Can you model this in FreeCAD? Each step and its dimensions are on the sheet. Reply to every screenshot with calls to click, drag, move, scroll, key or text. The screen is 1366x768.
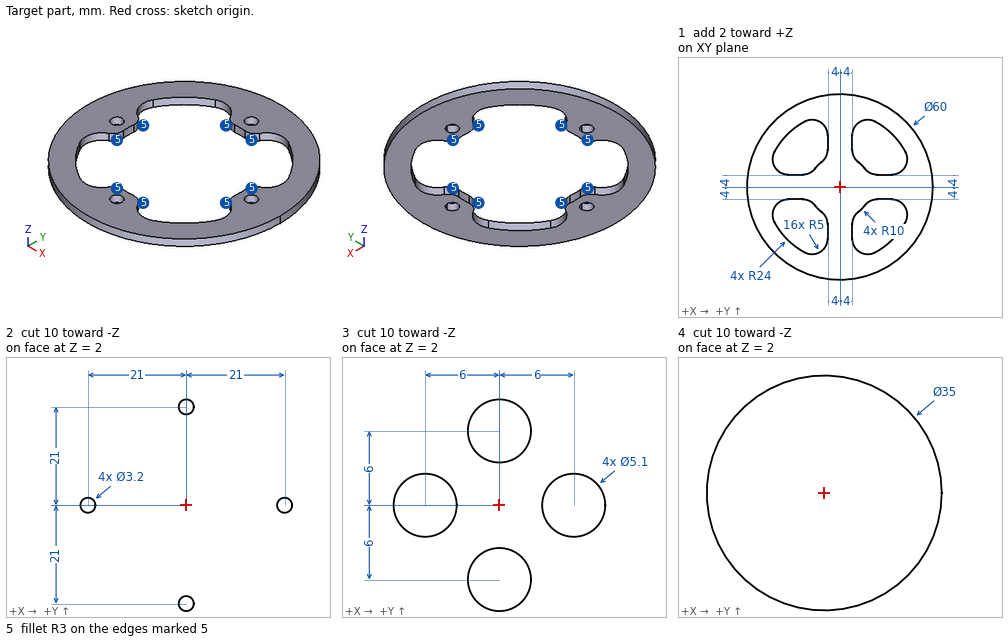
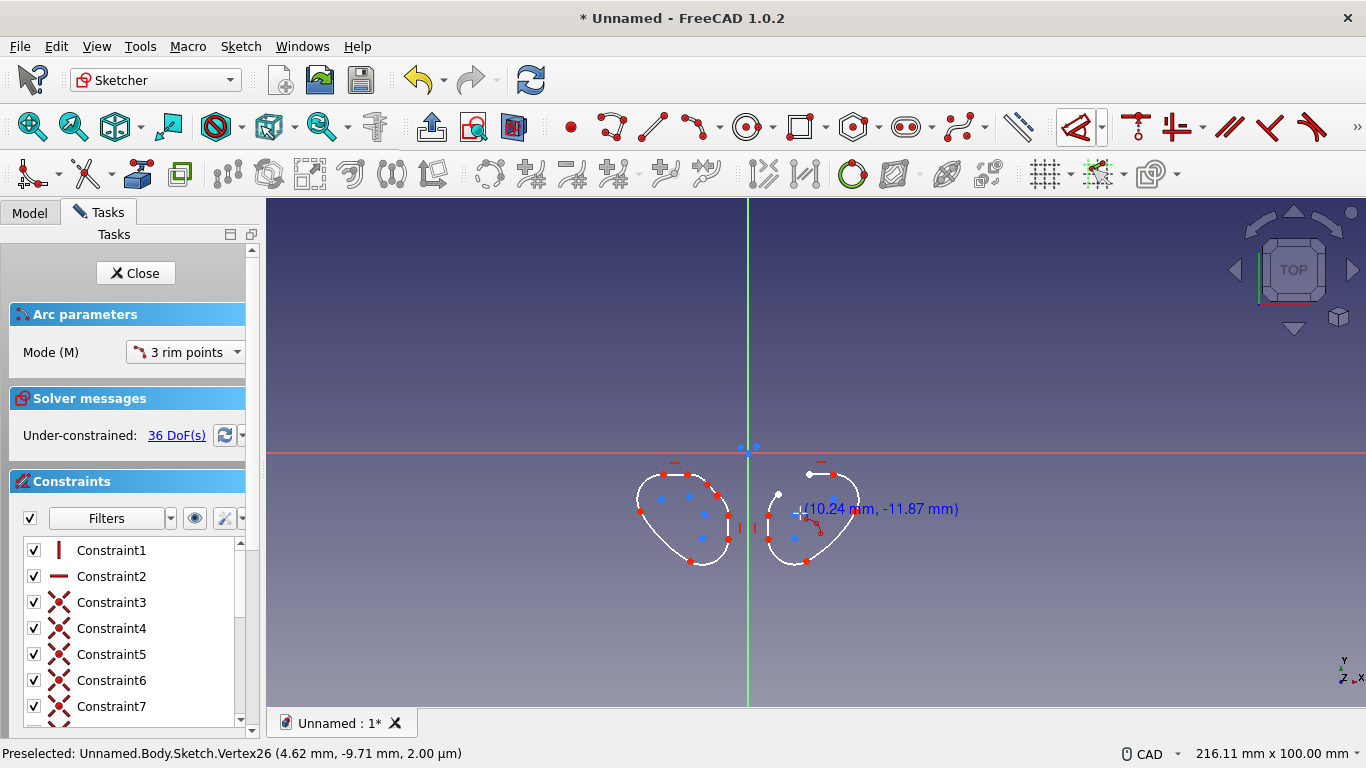
click(779, 494)
click(789, 484)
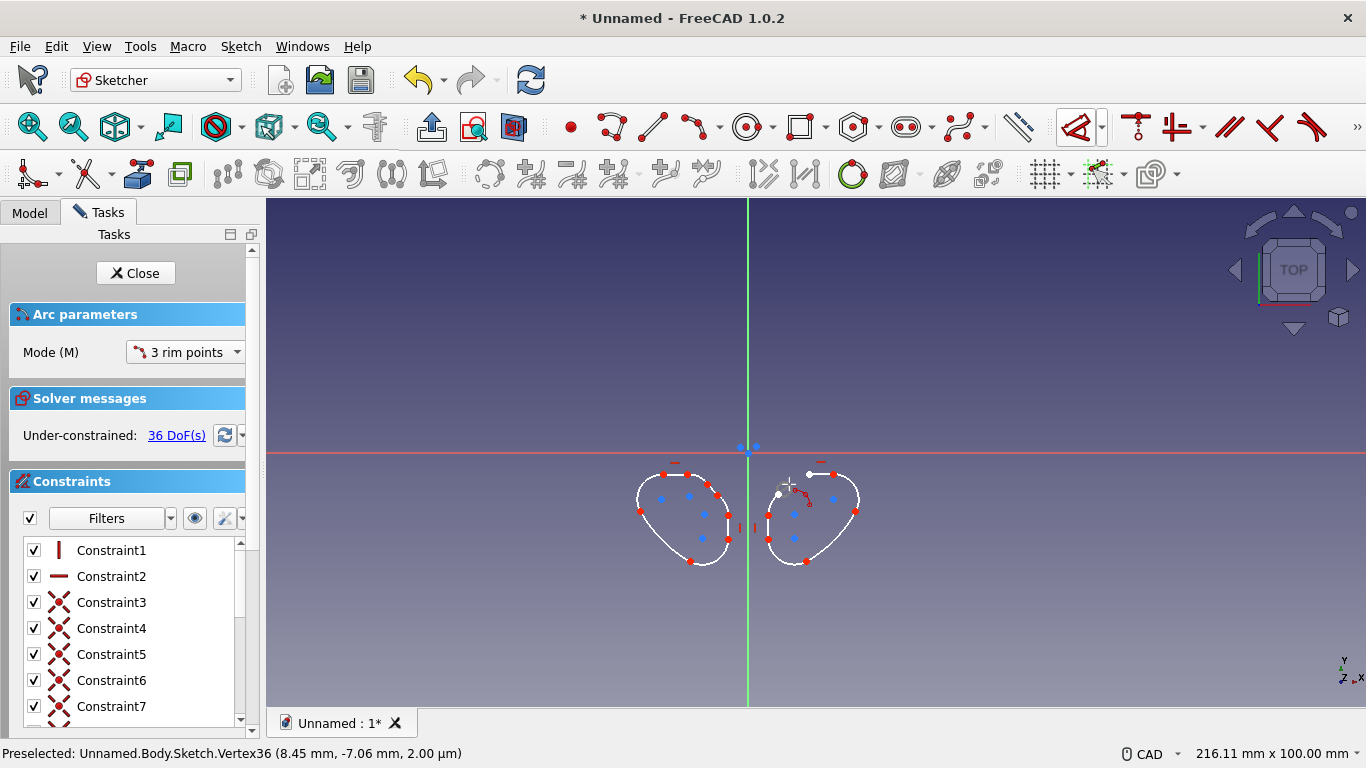
scroll(784, 489, up, 18)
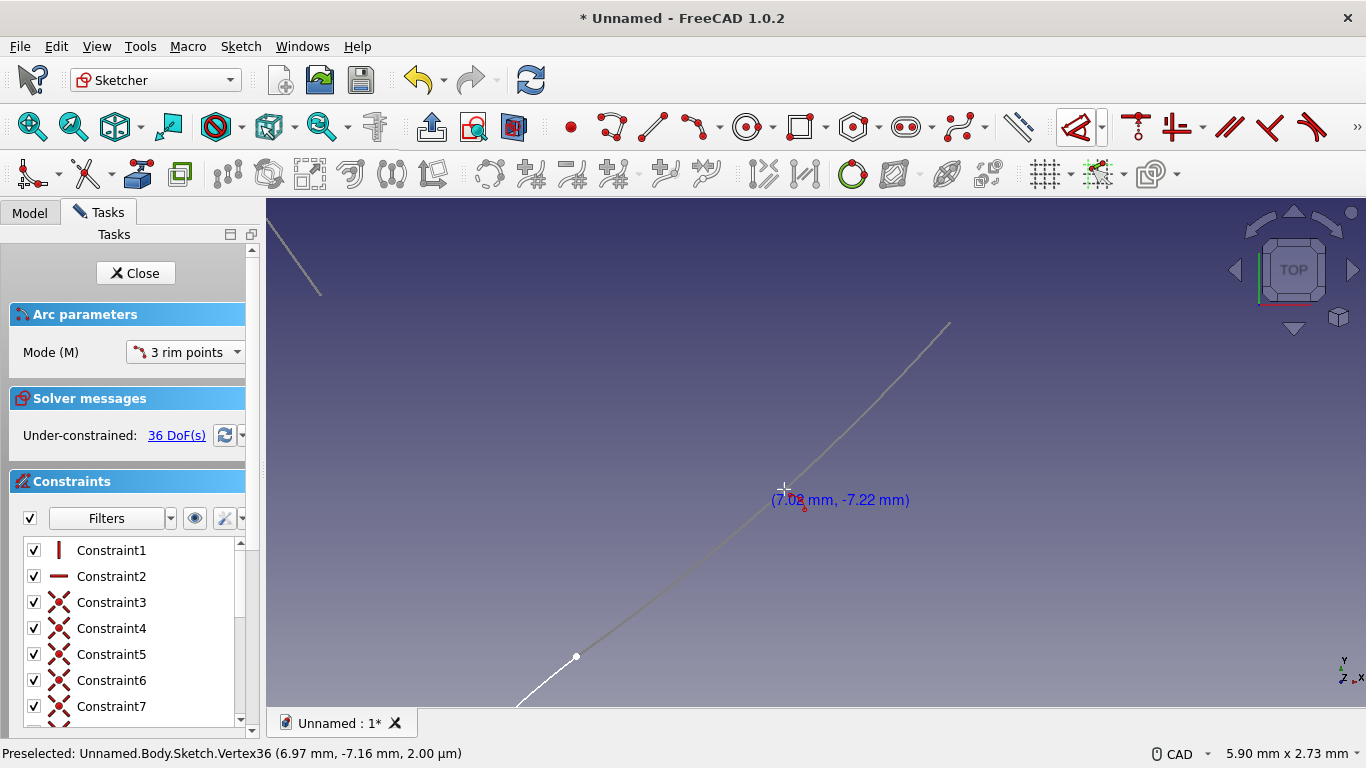
click(777, 477)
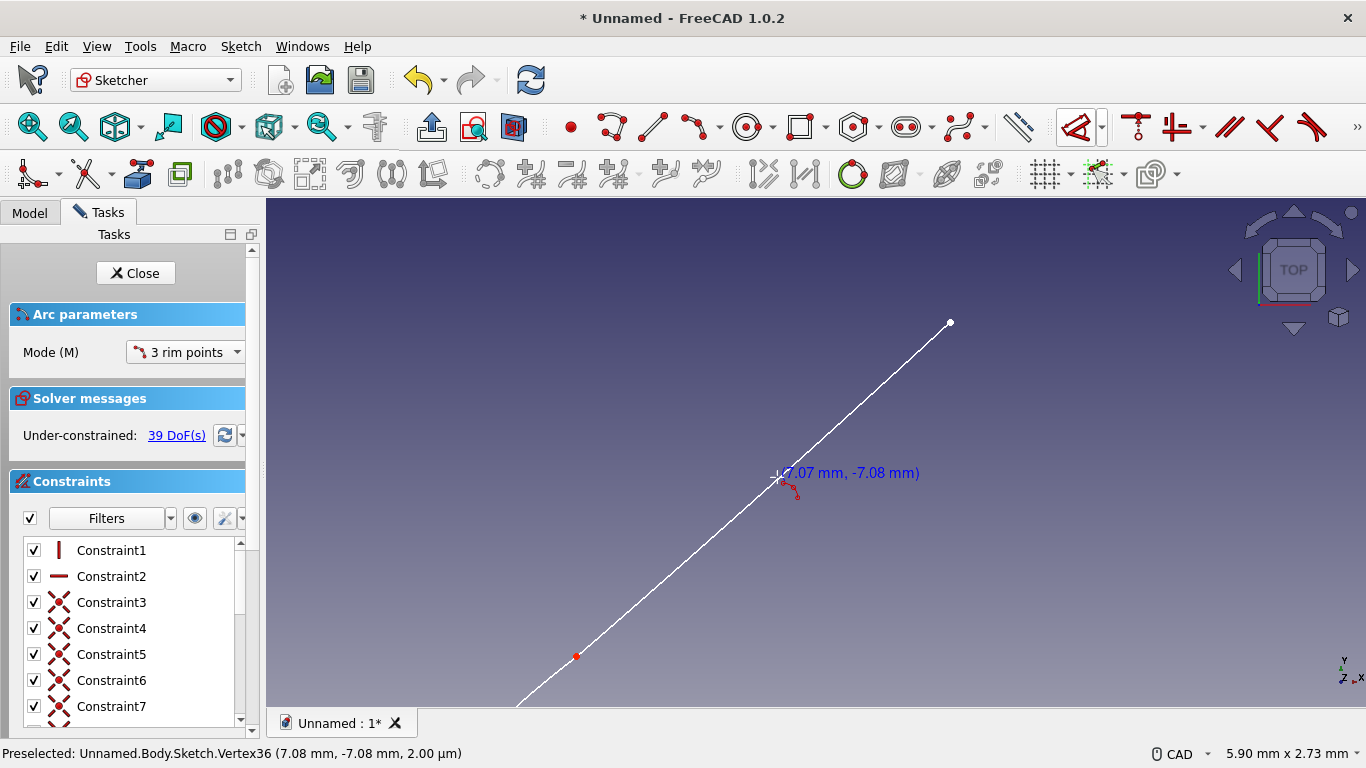
scroll(792, 497, down, 17)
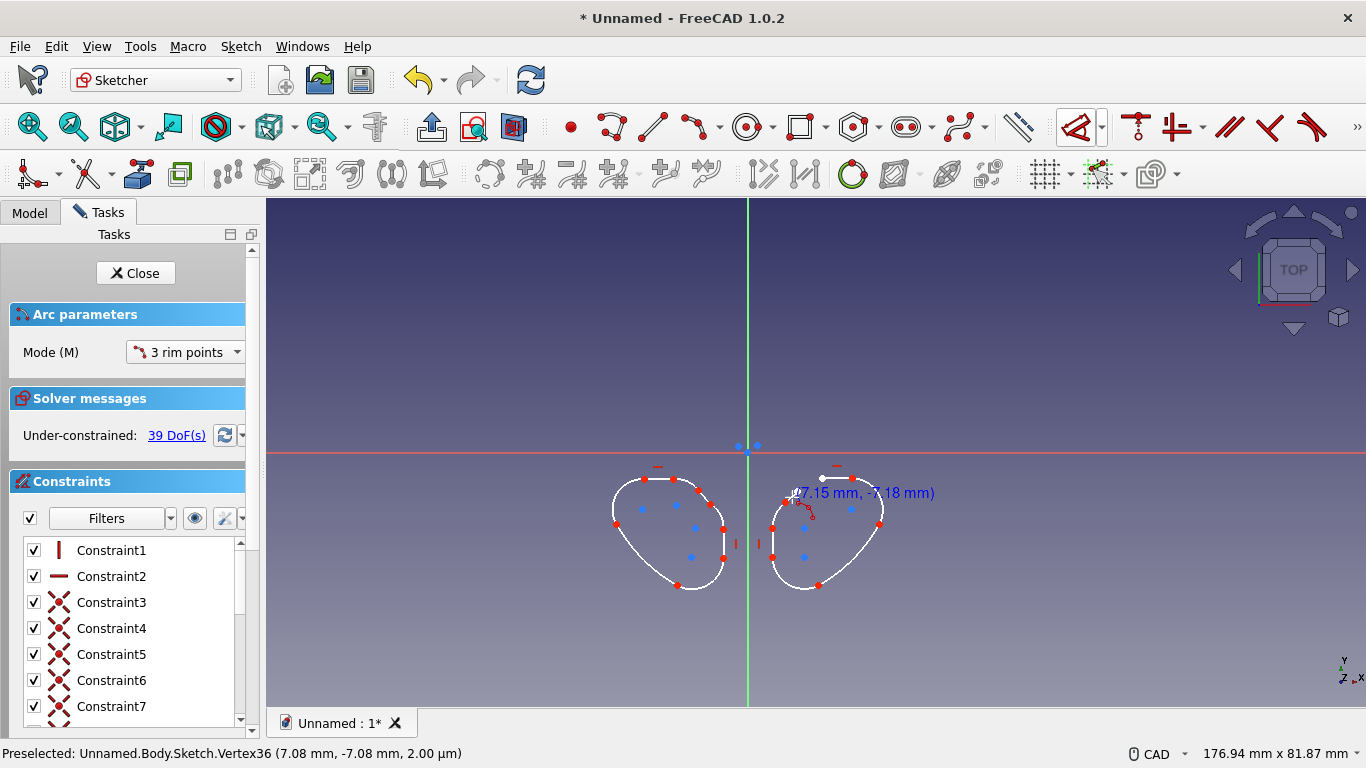
click(798, 492)
click(823, 478)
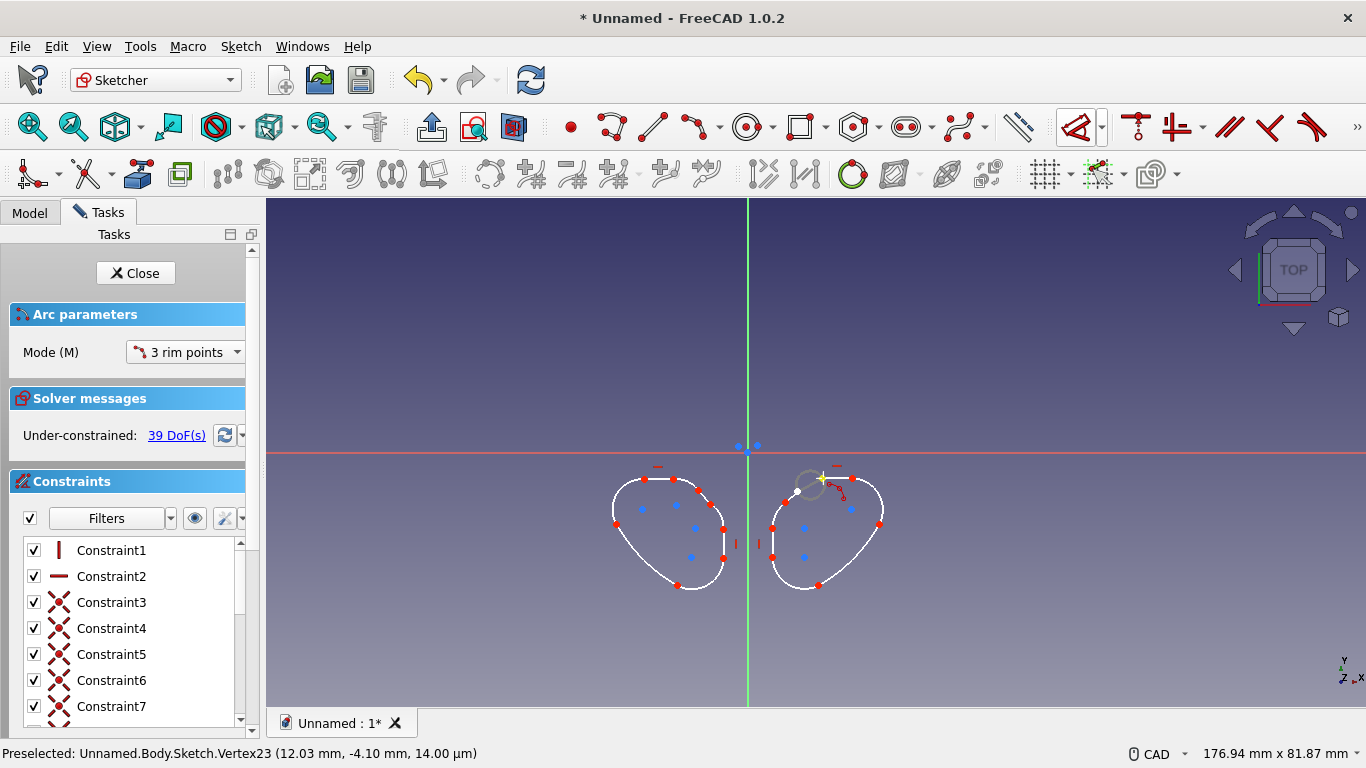
scroll(809, 481, up, 8)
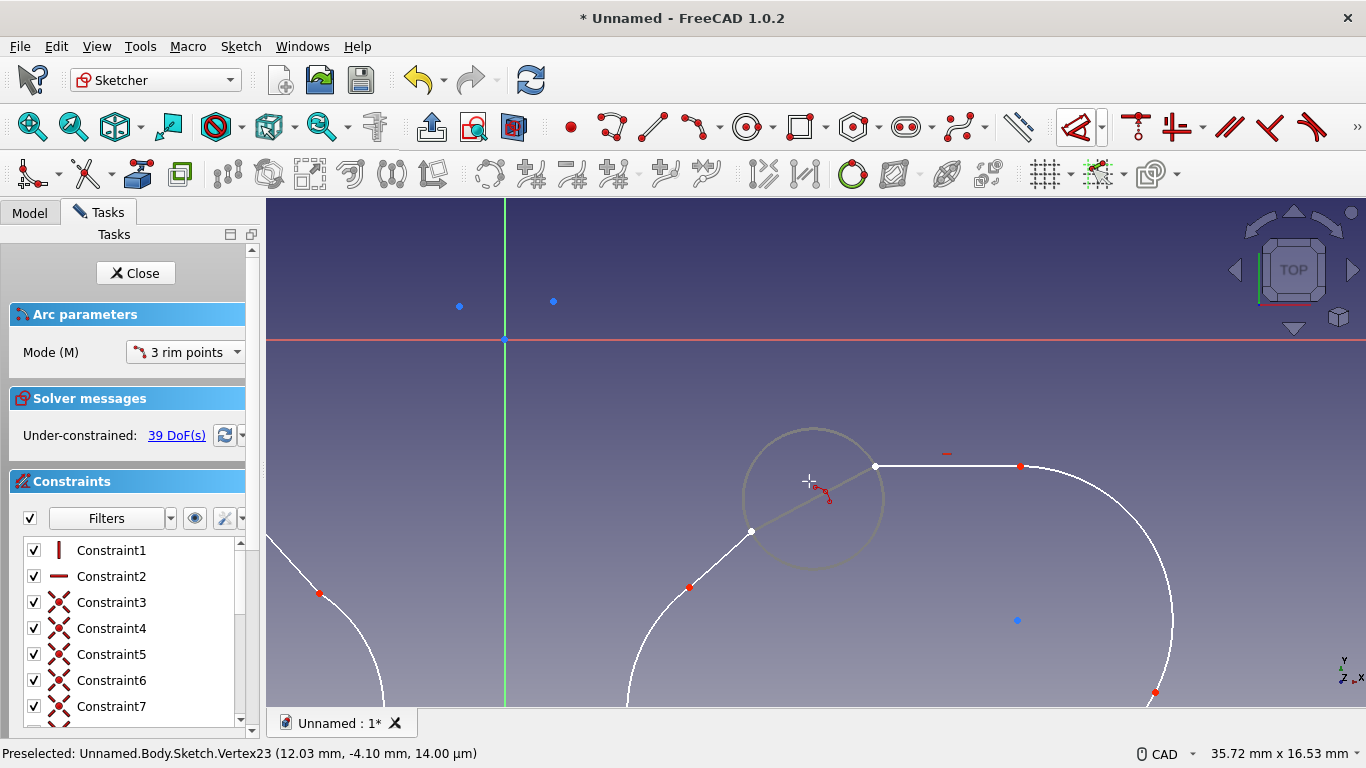
click(806, 479)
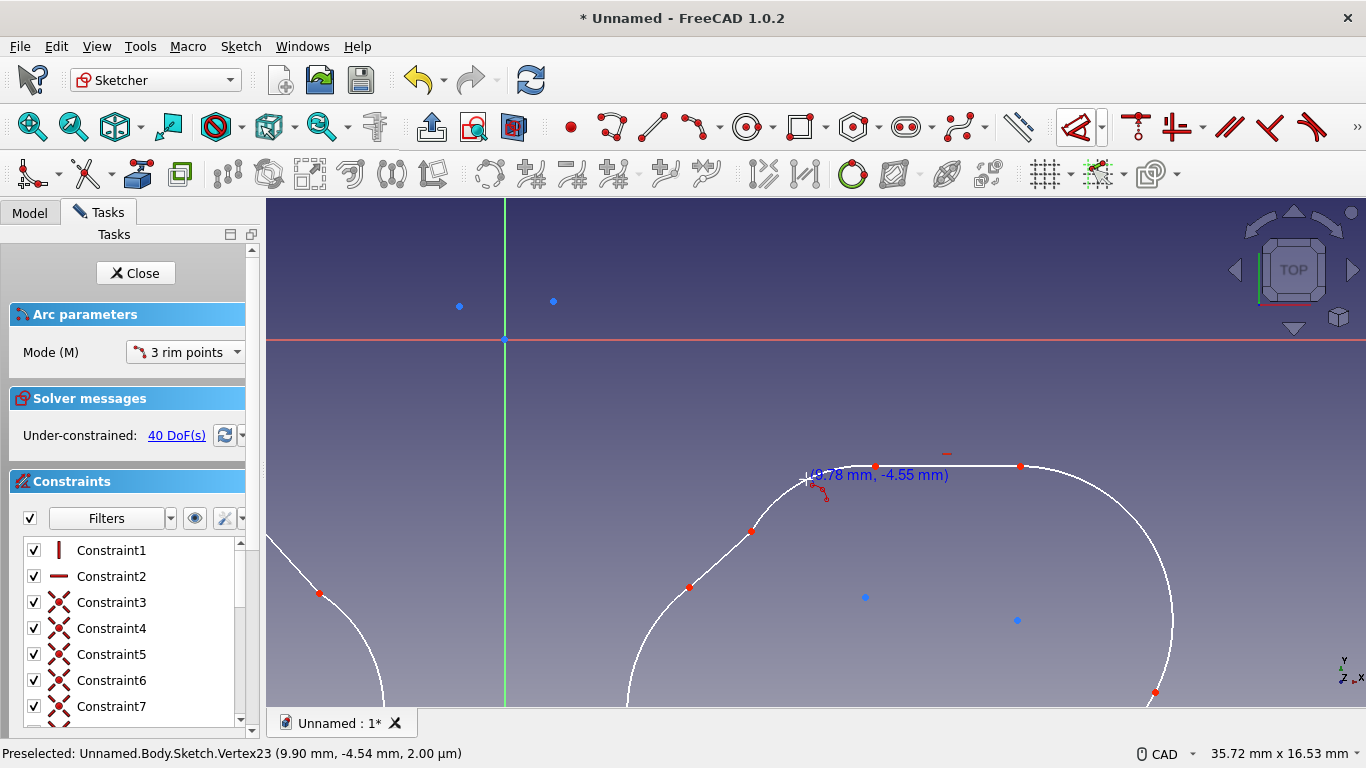
key(g)
key(l)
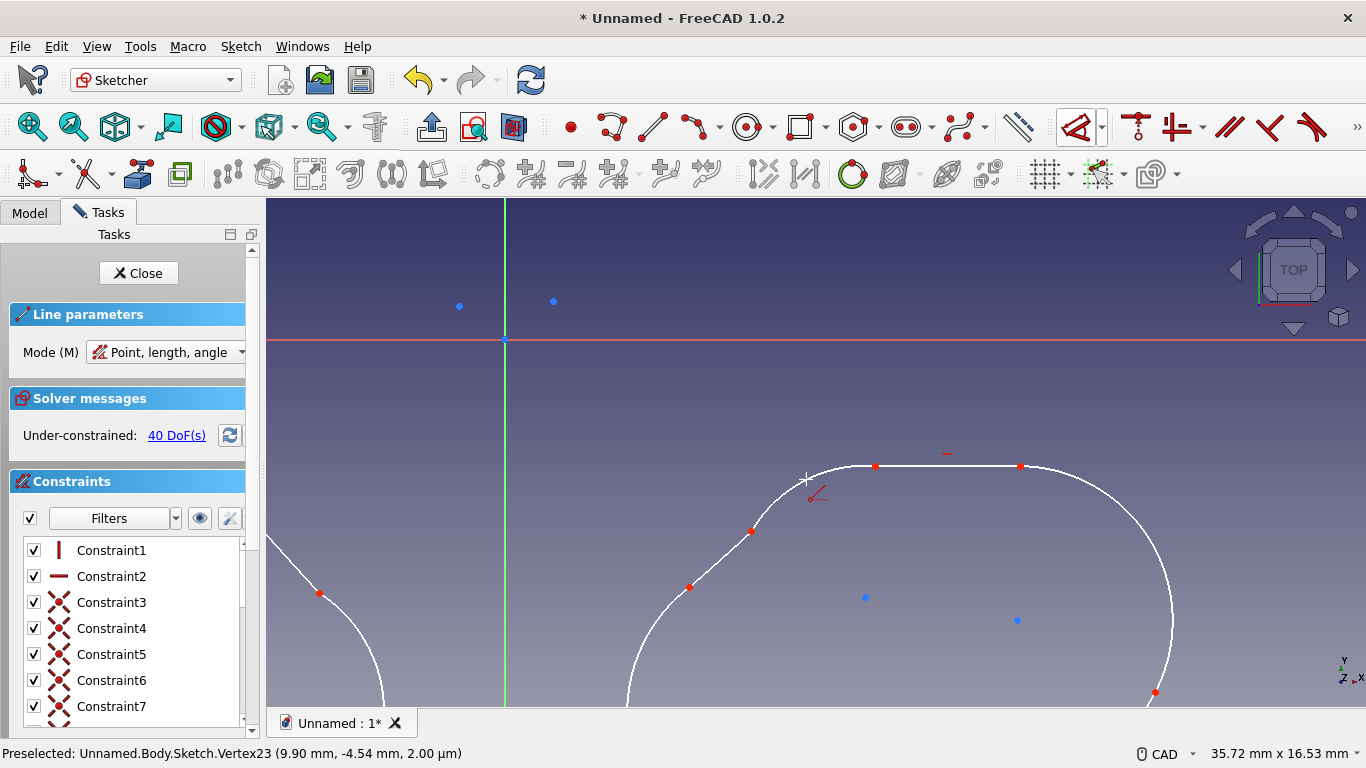
scroll(796, 475, down, 9)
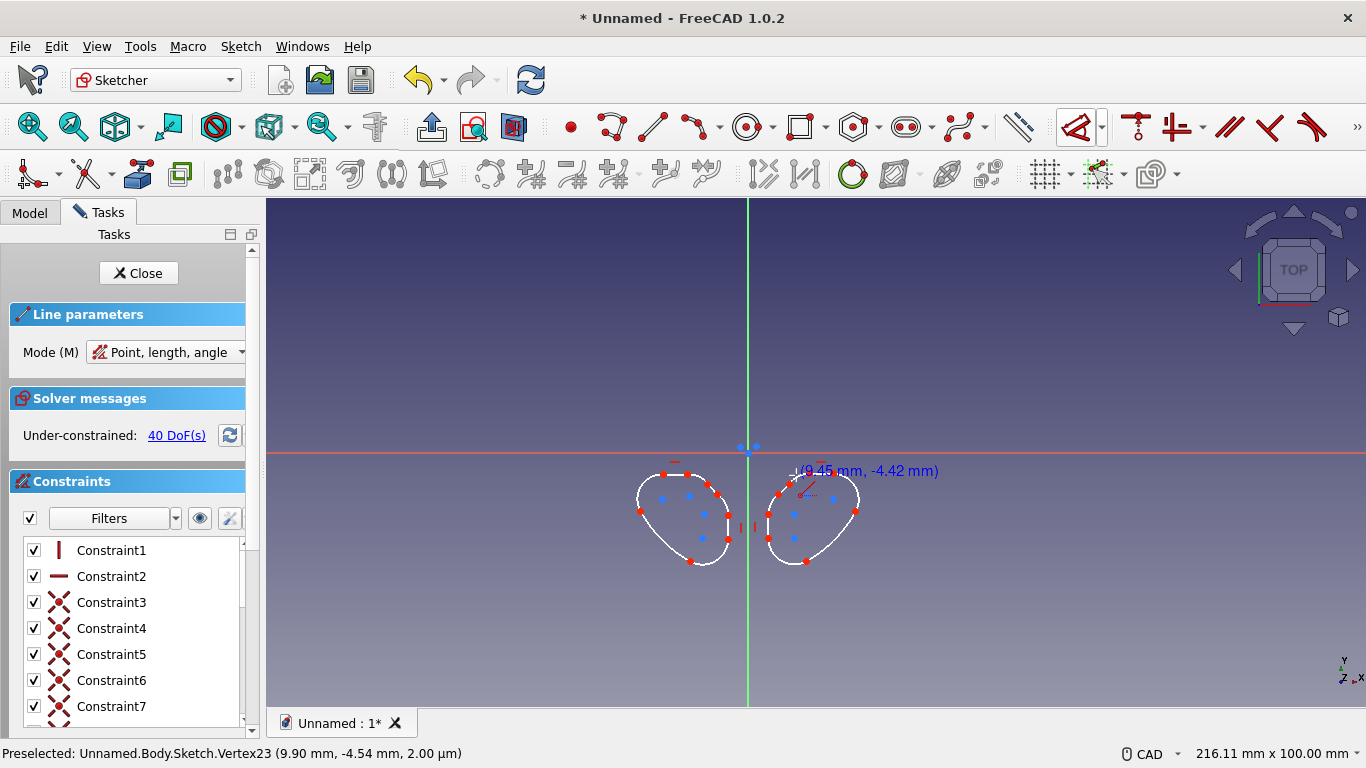
click(728, 368)
click(728, 392)